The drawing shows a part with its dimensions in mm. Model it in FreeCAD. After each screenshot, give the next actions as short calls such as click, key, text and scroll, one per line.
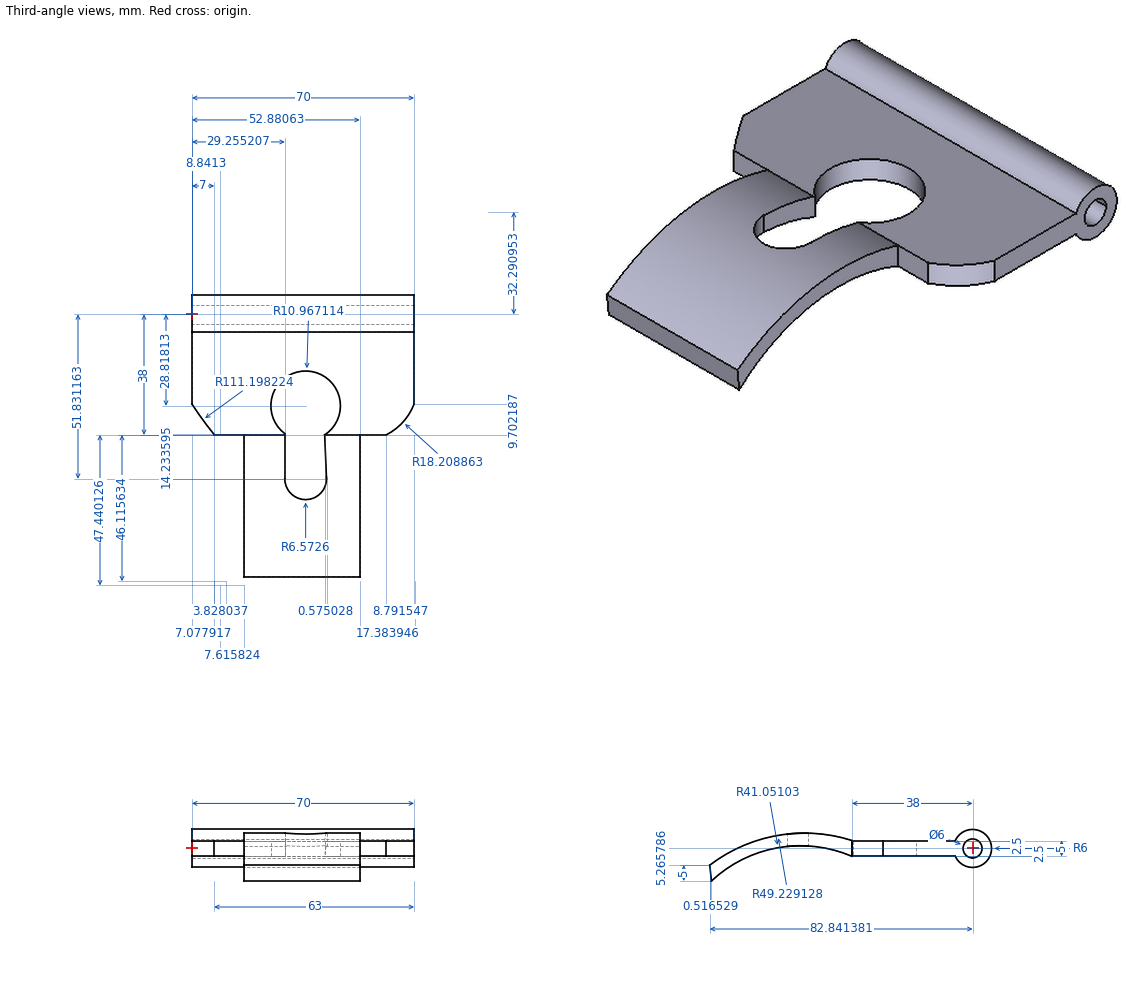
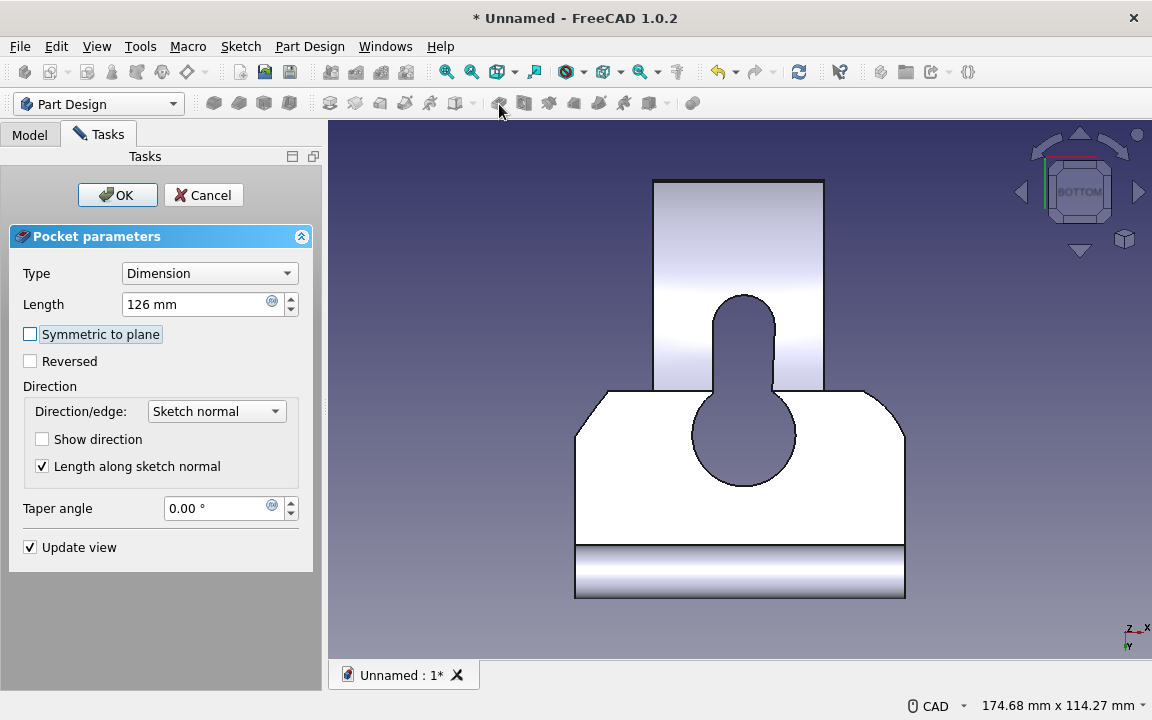
click(31, 334)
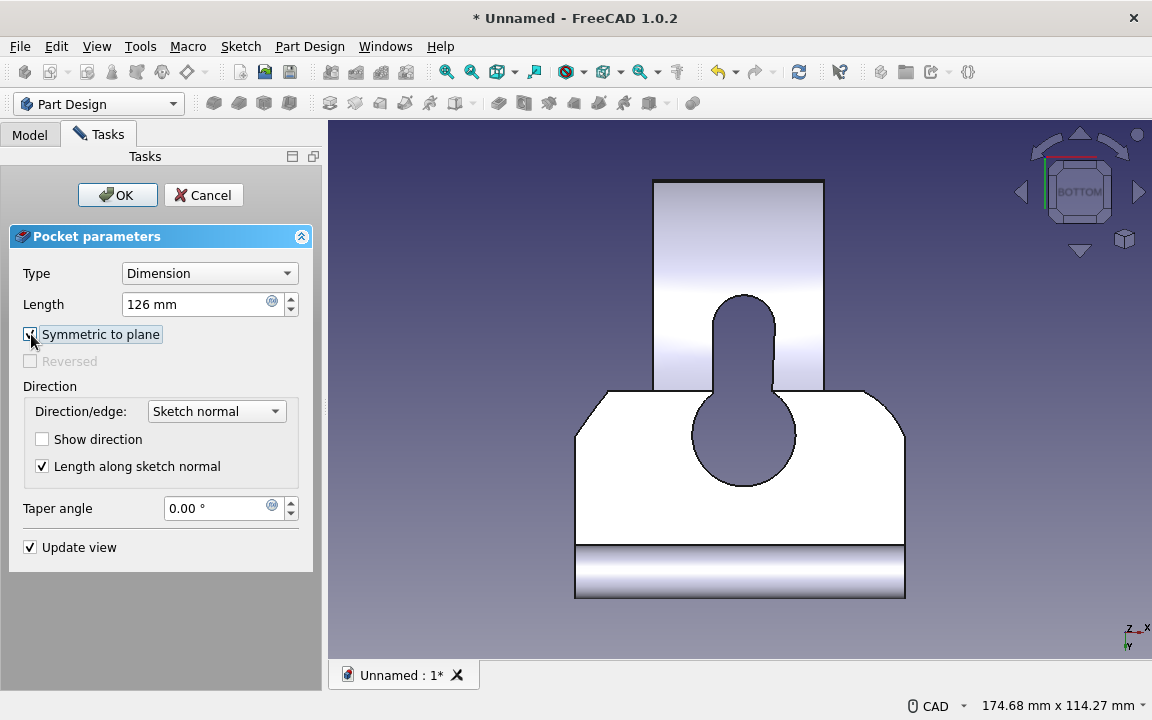
click(118, 195)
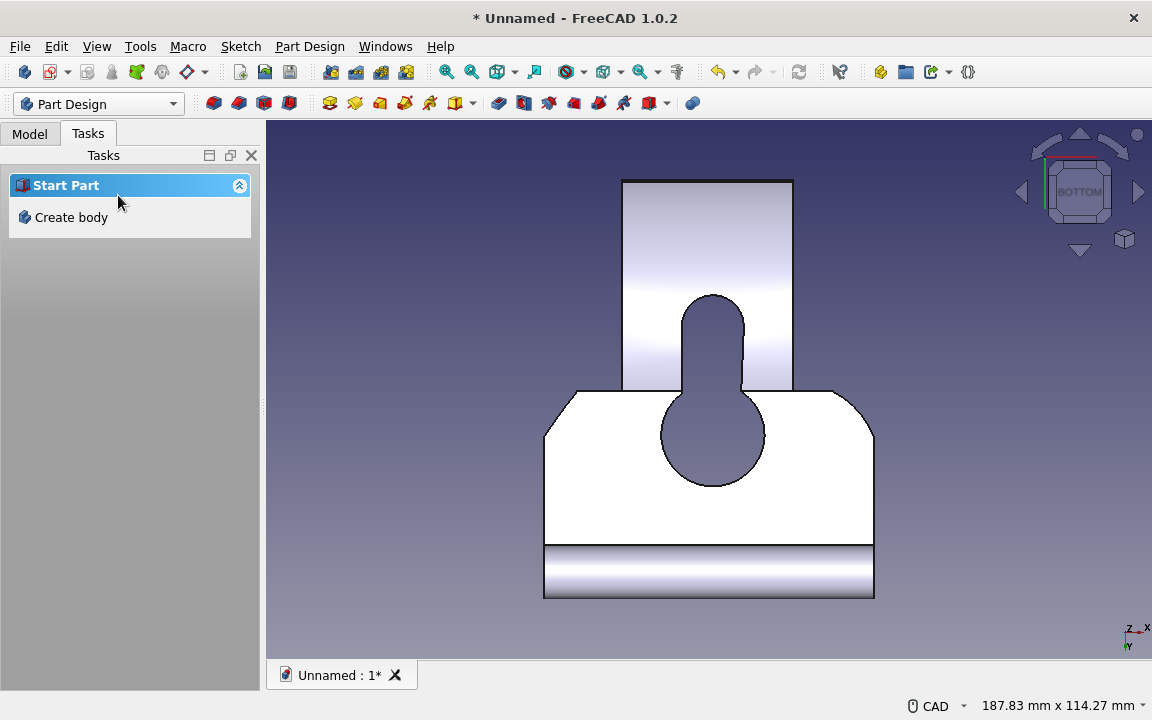
key(0)